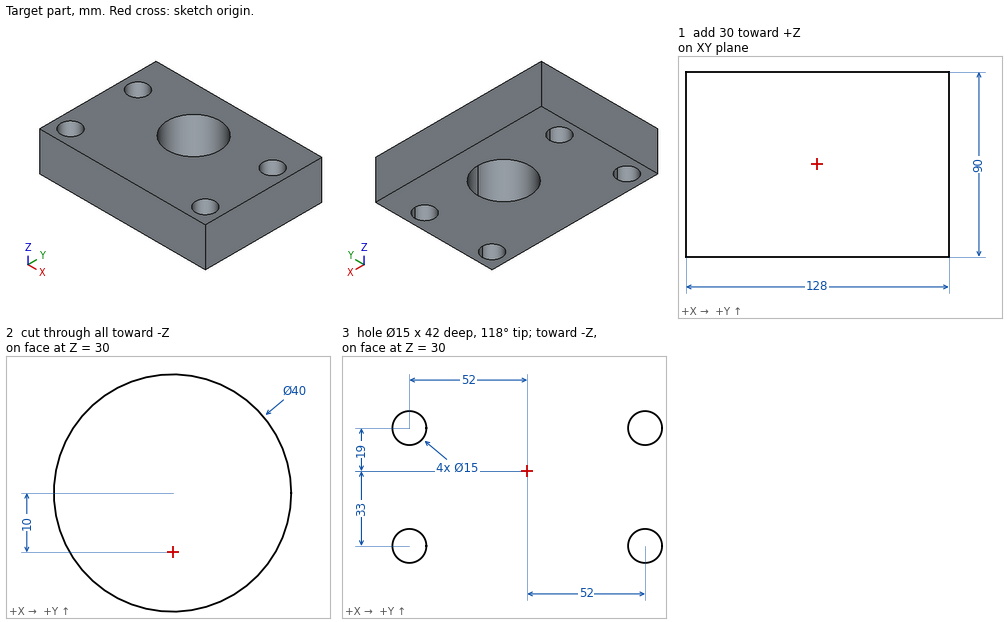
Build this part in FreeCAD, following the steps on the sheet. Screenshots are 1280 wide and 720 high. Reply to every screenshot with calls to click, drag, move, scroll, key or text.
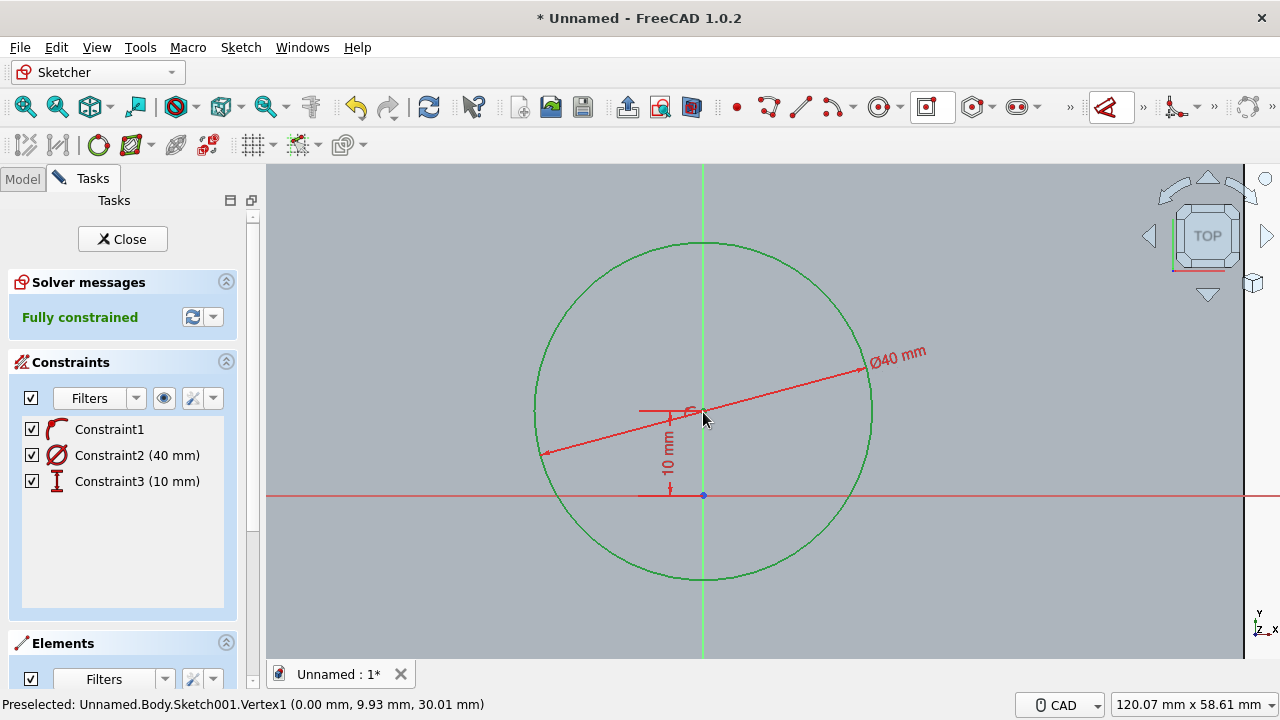
click(123, 239)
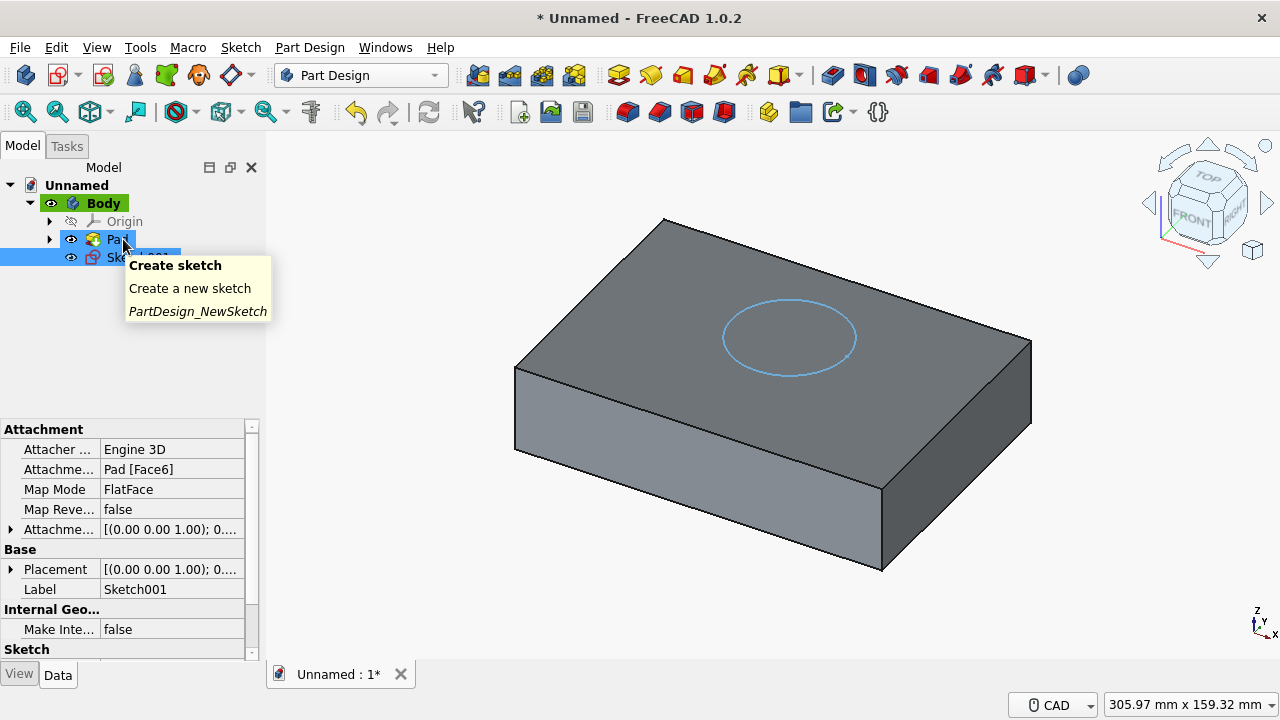
click(834, 76)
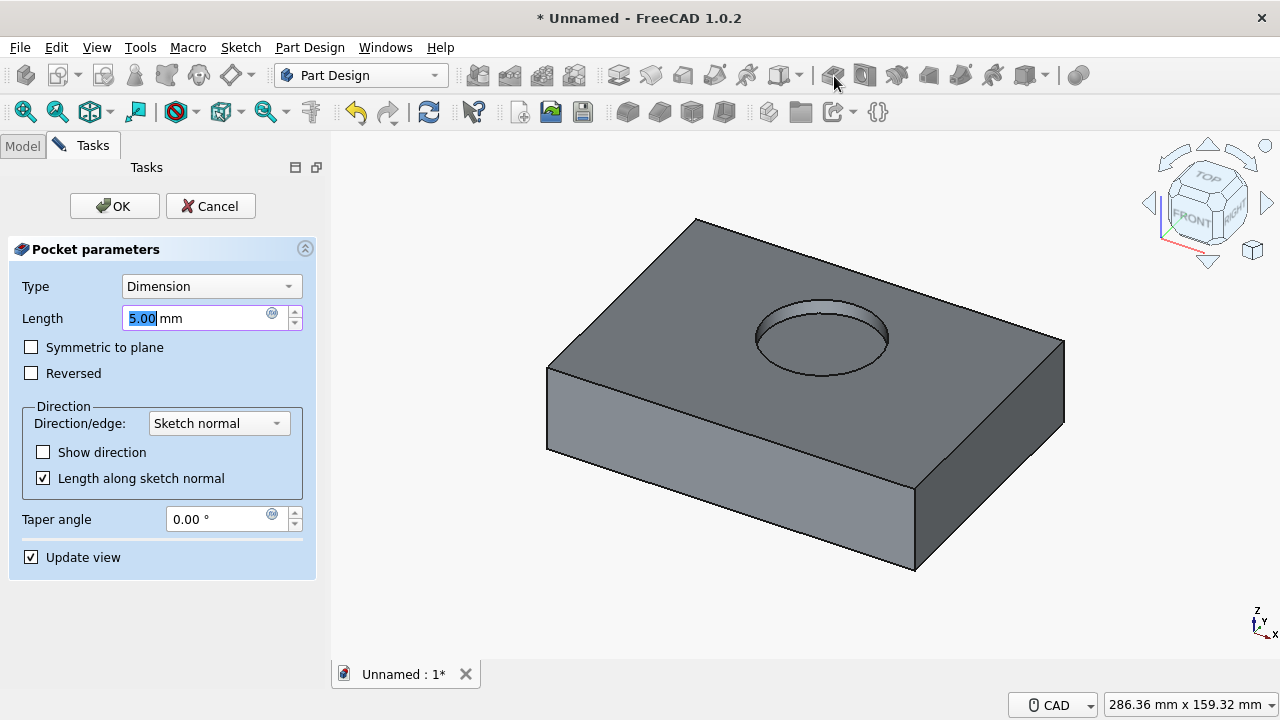
click(212, 286)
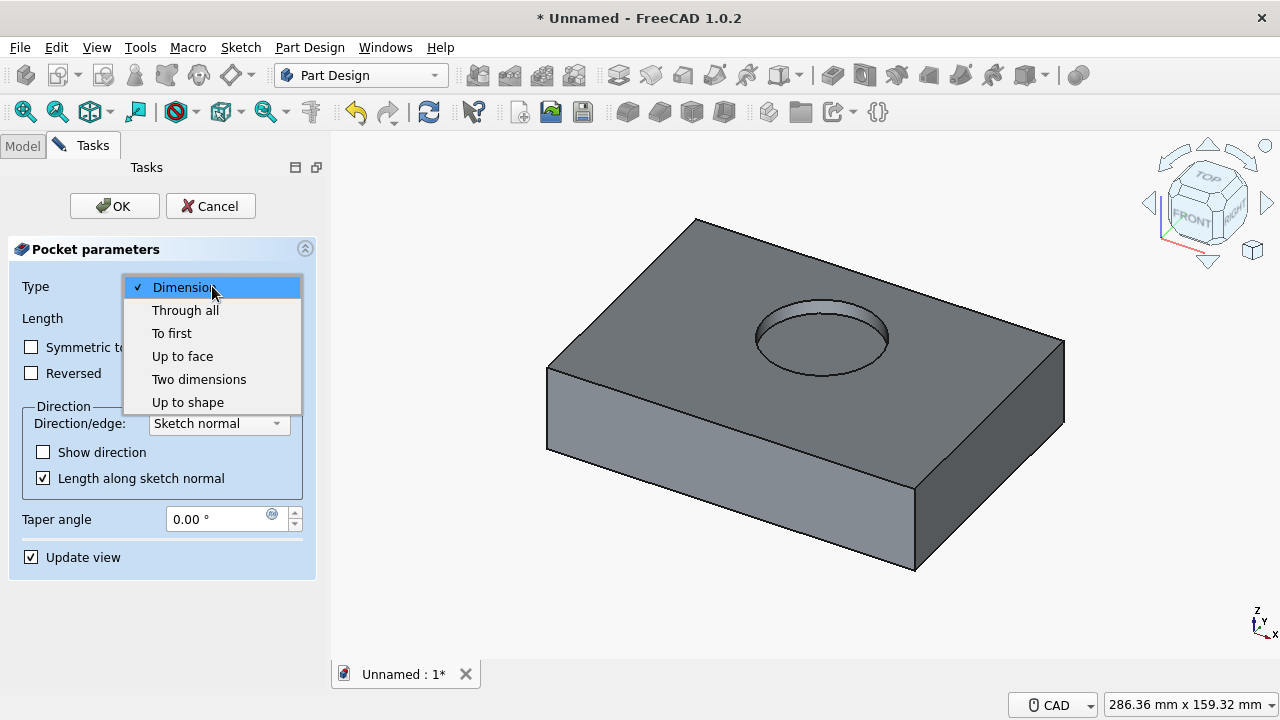
click(212, 310)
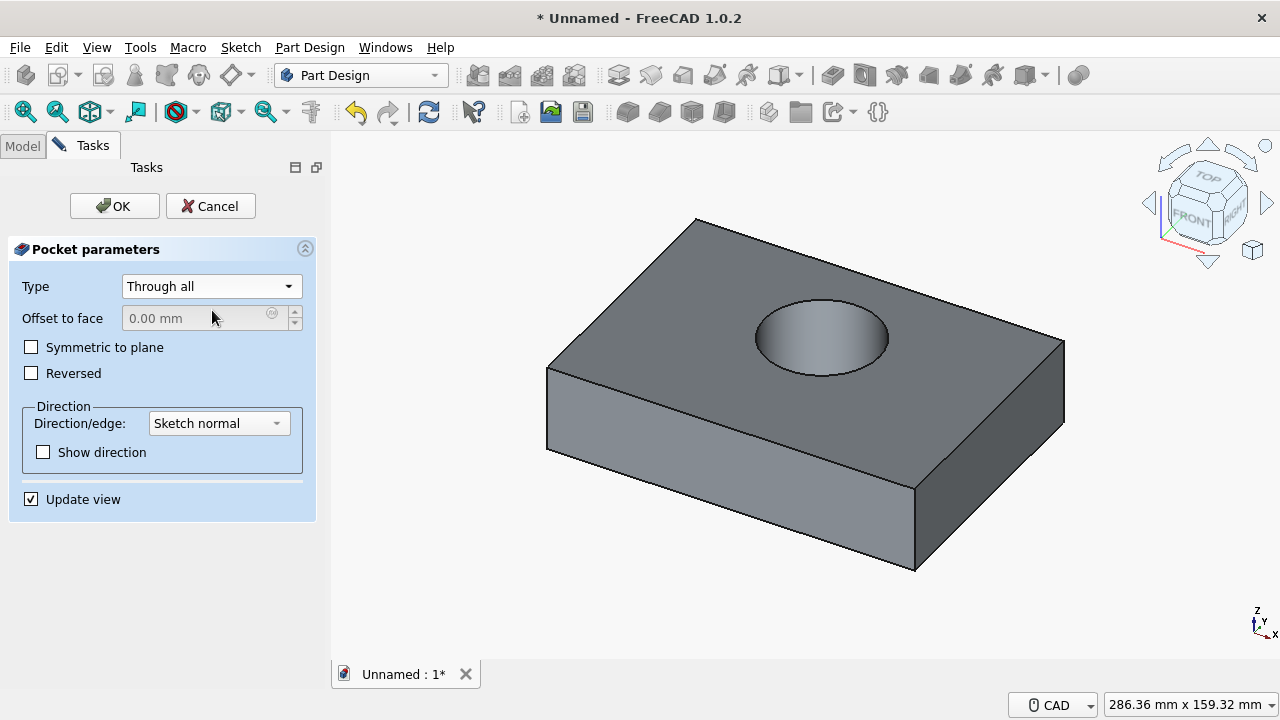
click(115, 206)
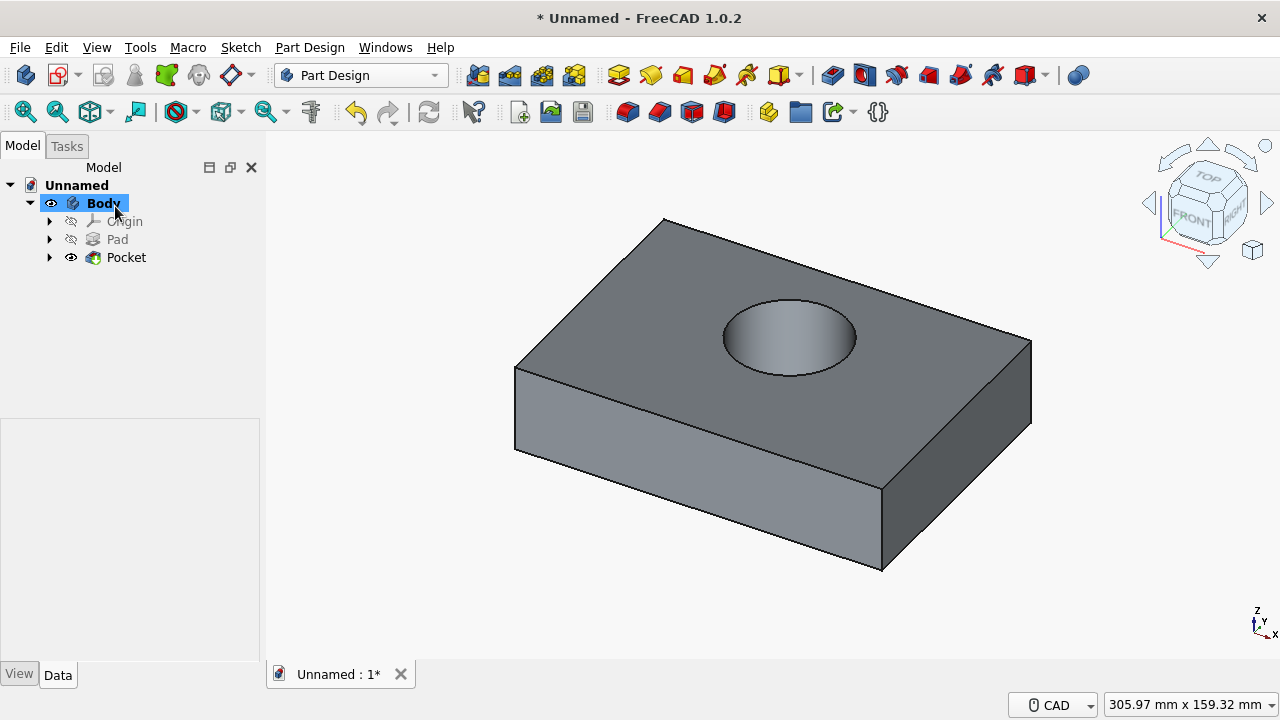
click(857, 409)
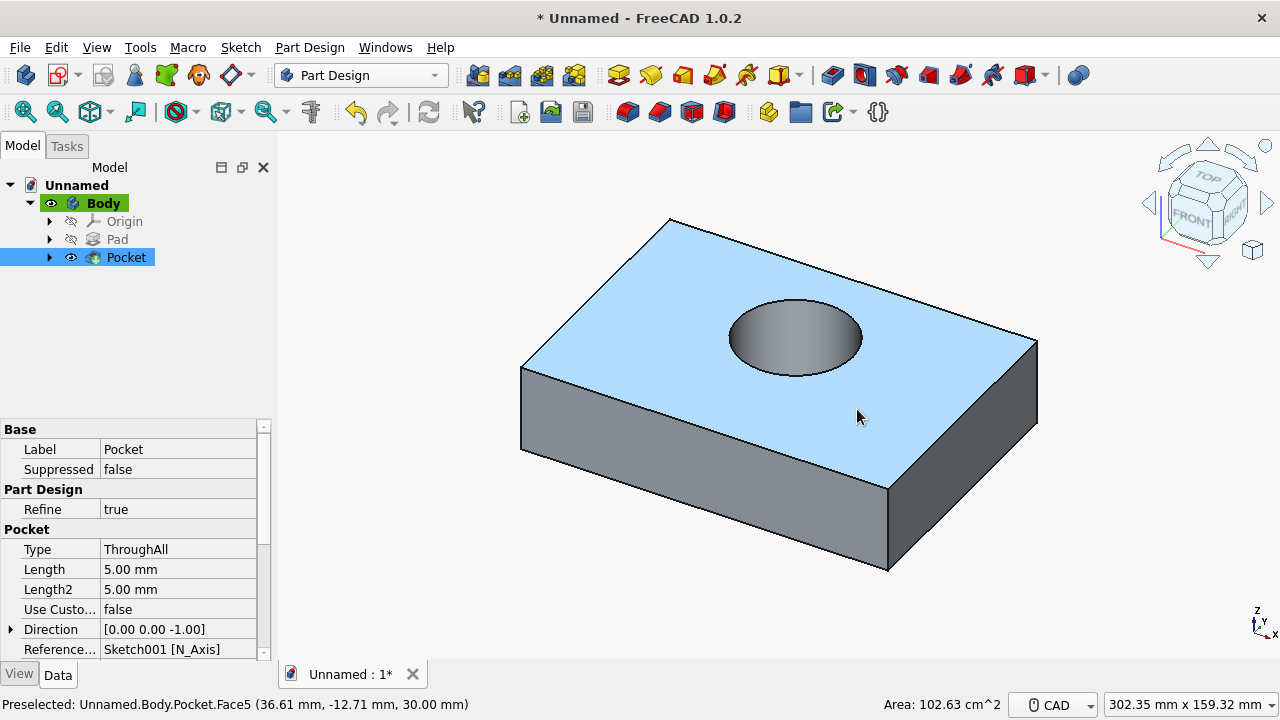
click(58, 76)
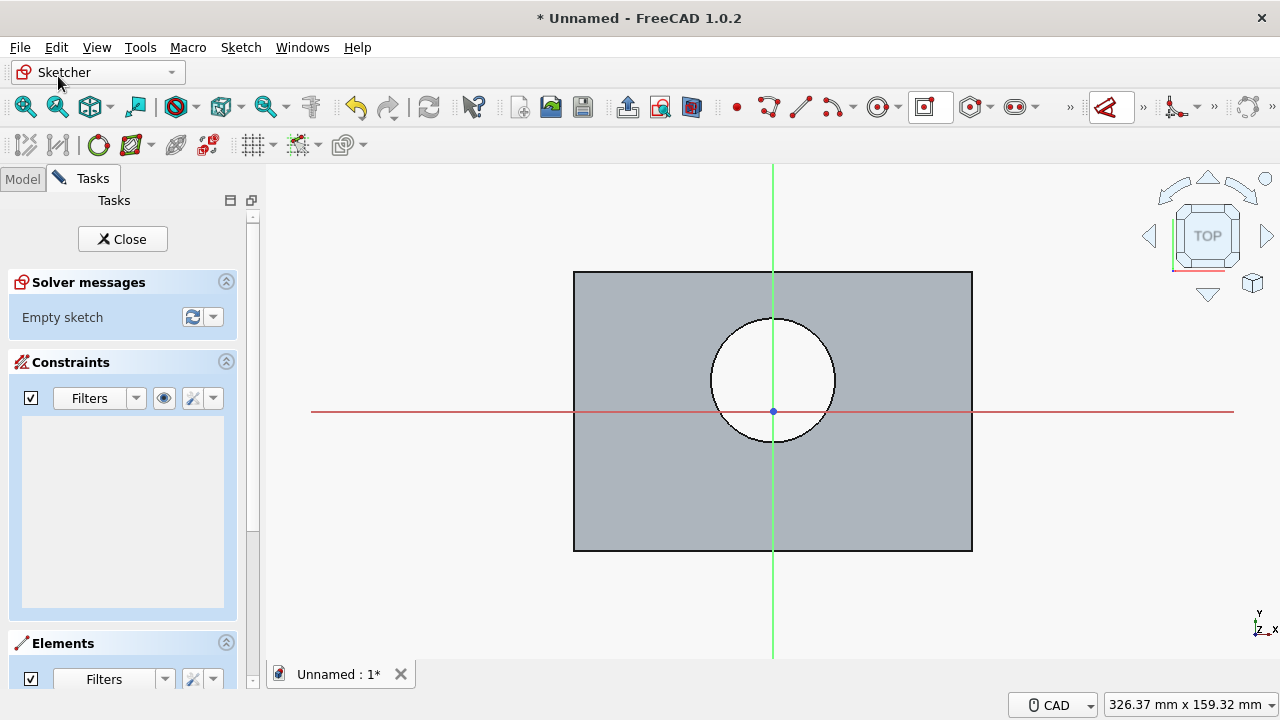
scroll(912, 477, up, 2)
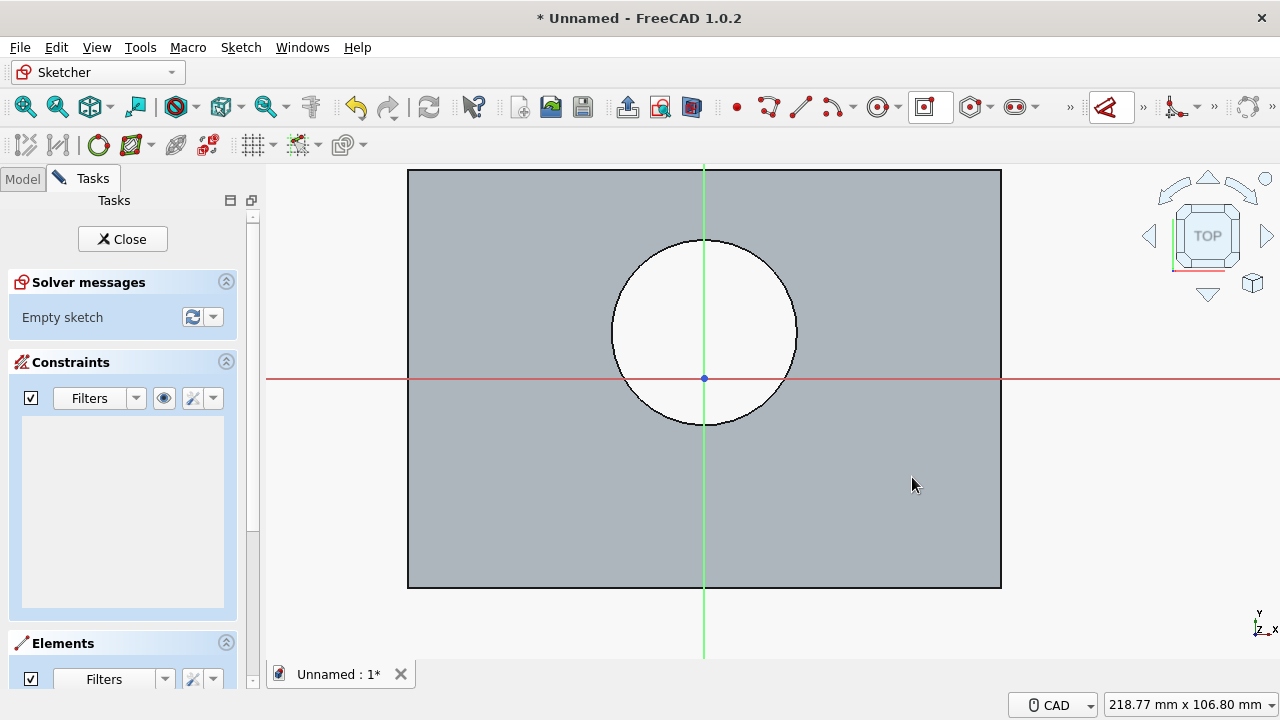
click(878, 108)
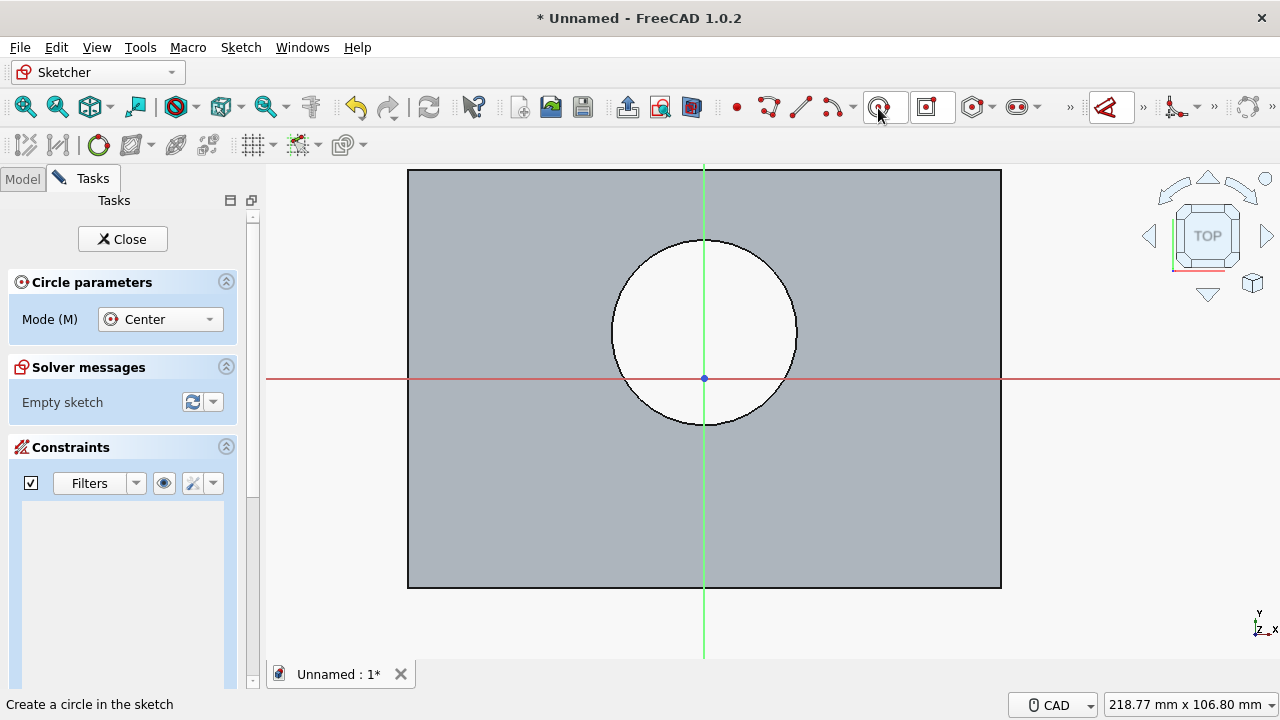
click(463, 291)
click(488, 266)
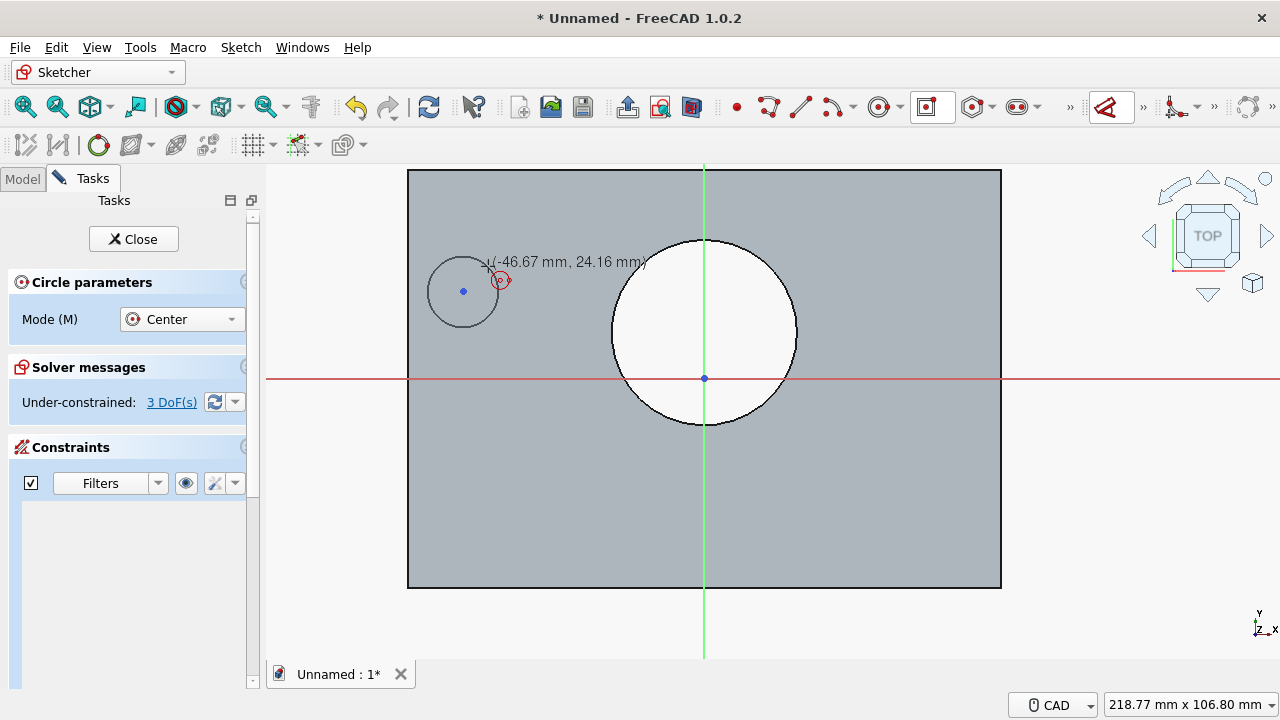
click(463, 532)
click(488, 507)